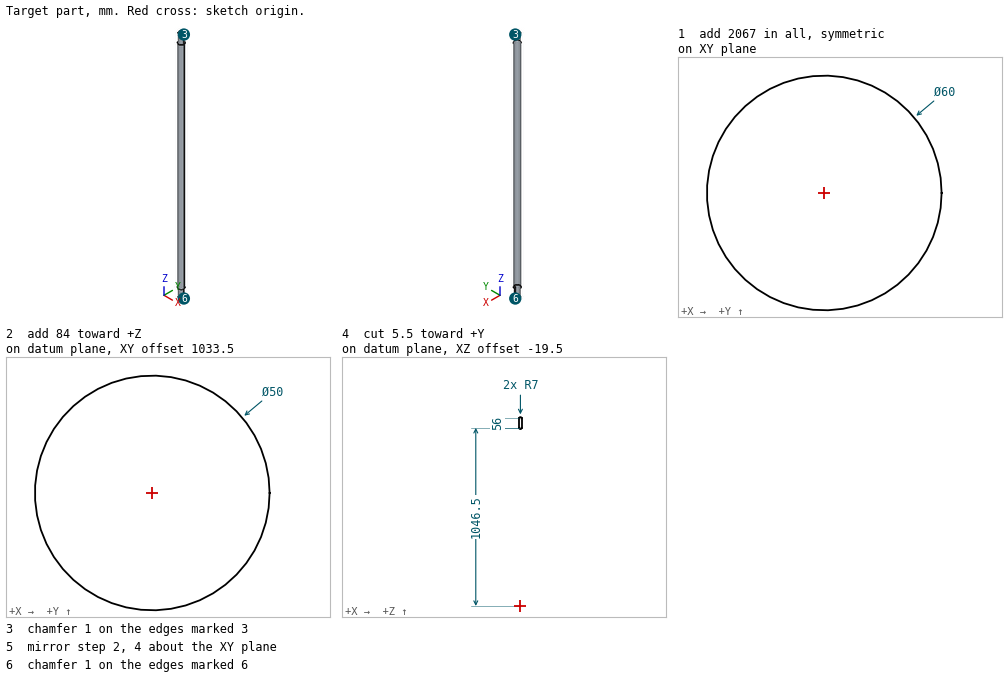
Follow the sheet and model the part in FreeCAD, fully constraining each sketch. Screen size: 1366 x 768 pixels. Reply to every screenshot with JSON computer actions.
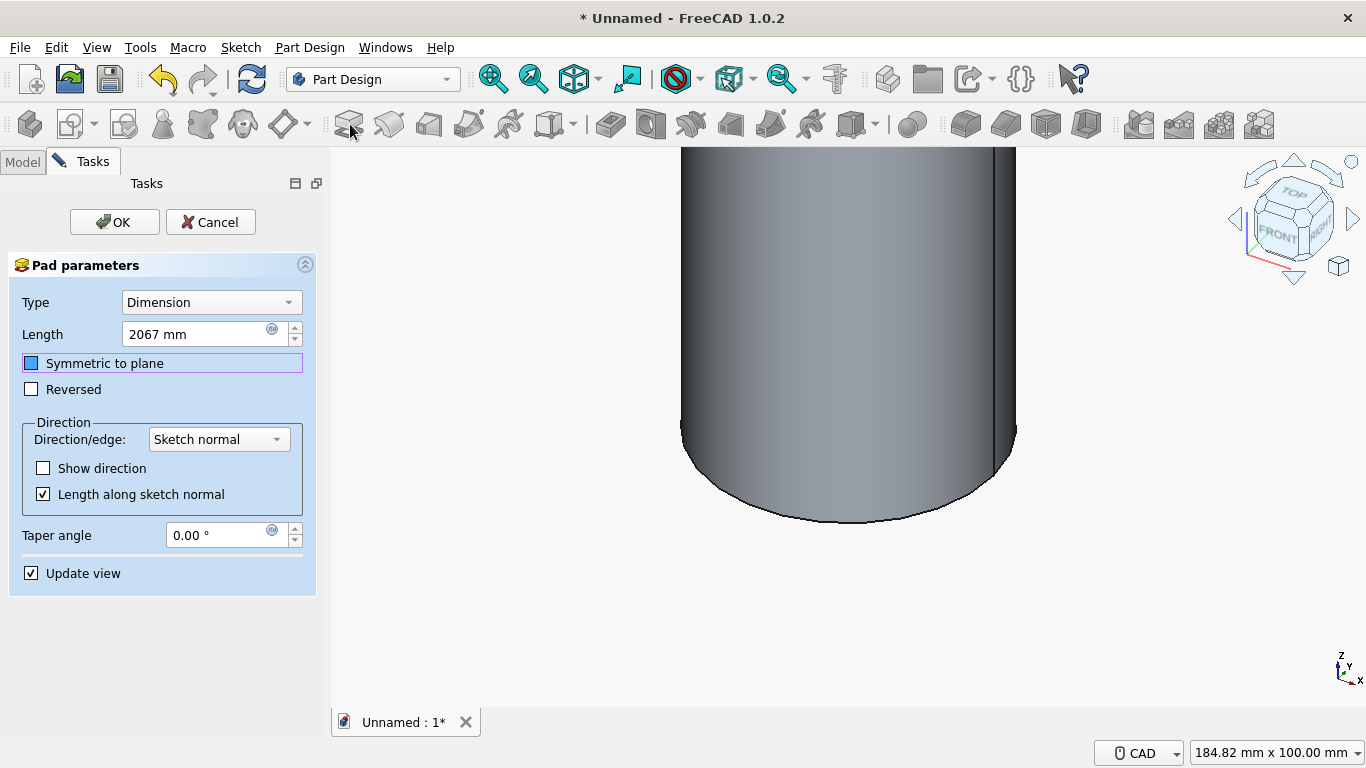
{"action": "left_click", "coordinate": [30, 363]}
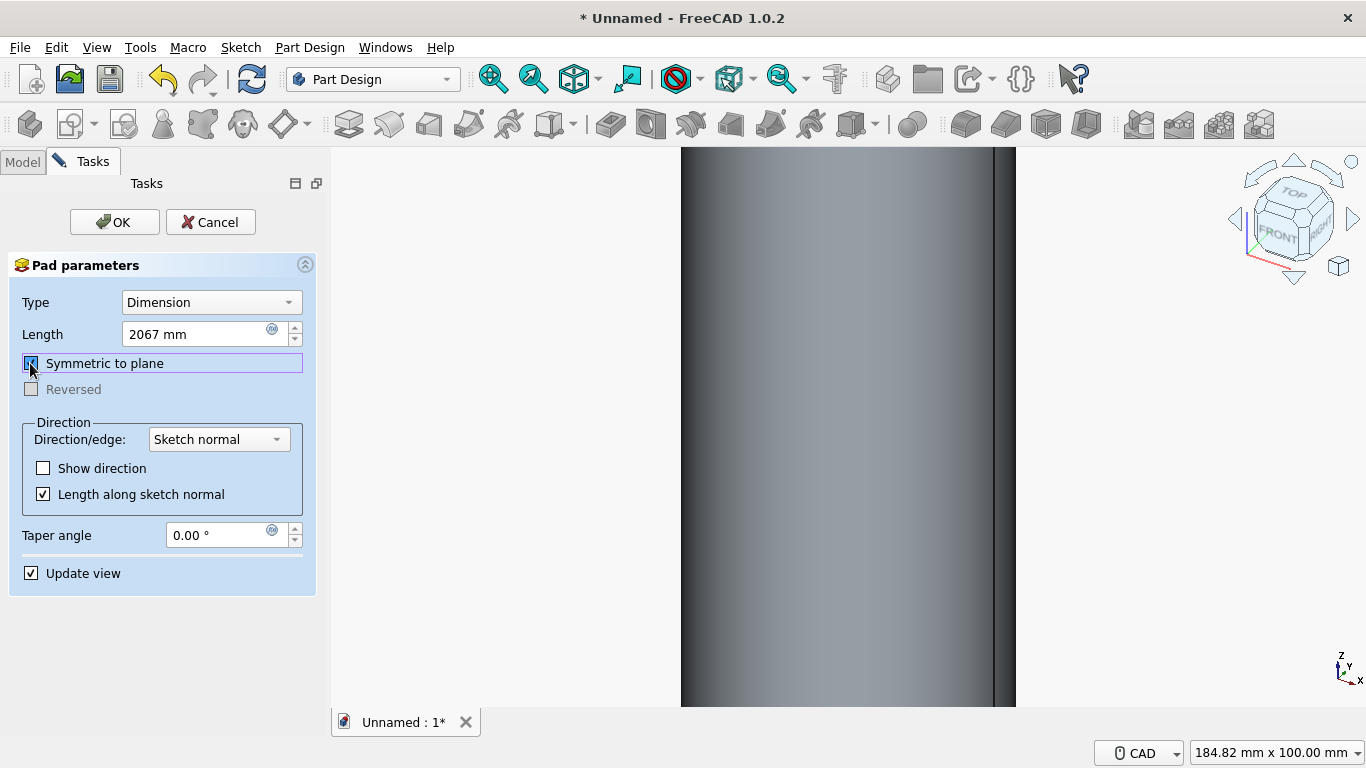
{"action": "left_click", "coordinate": [115, 222]}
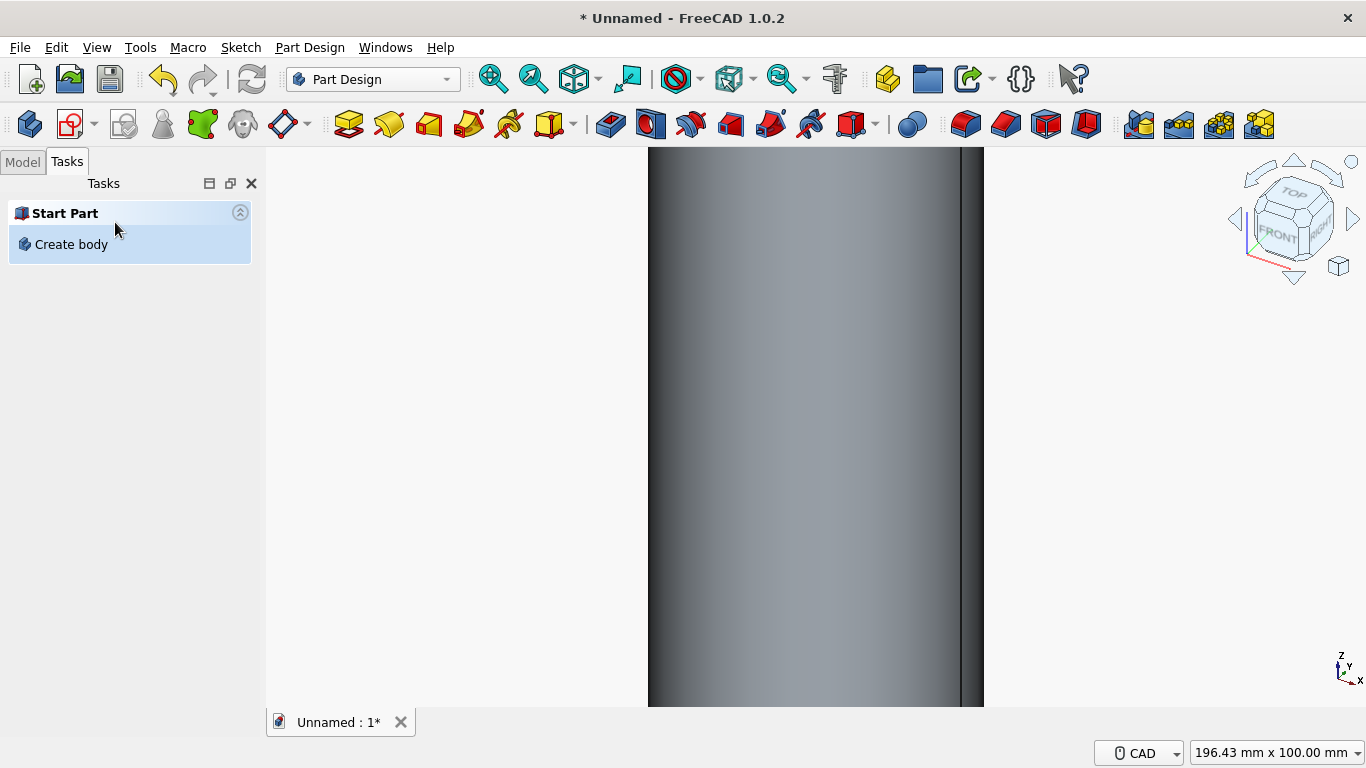
{"action": "left_click", "coordinate": [494, 80]}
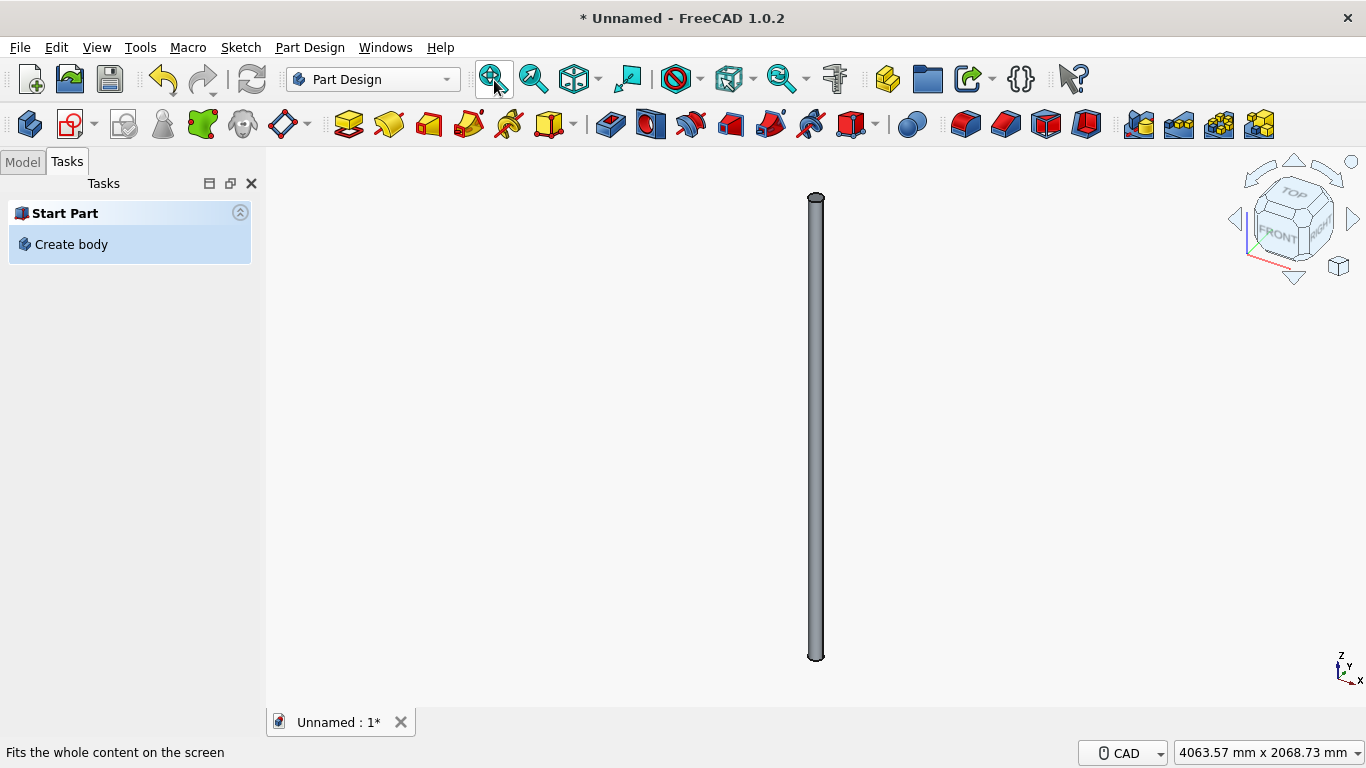
{"action": "key", "text": "0"}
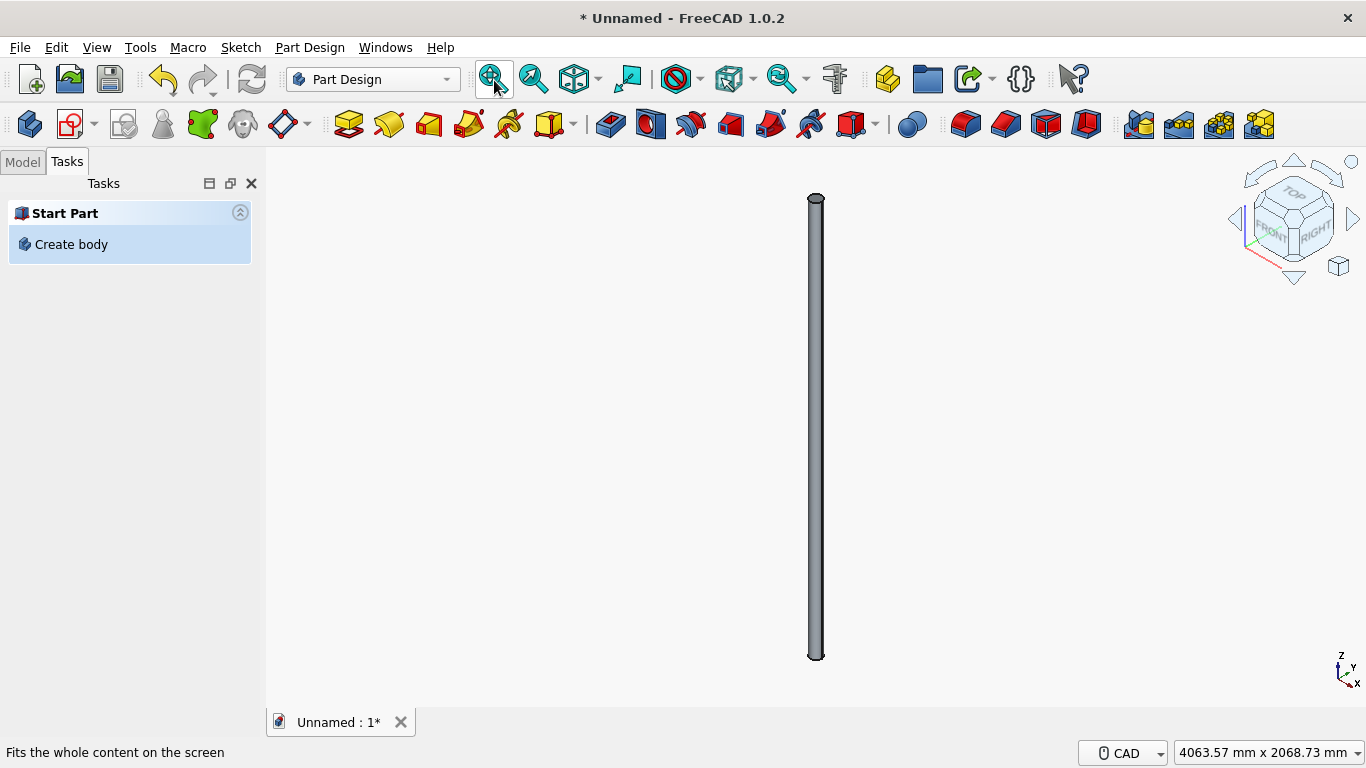
{"action": "key", "text": "2"}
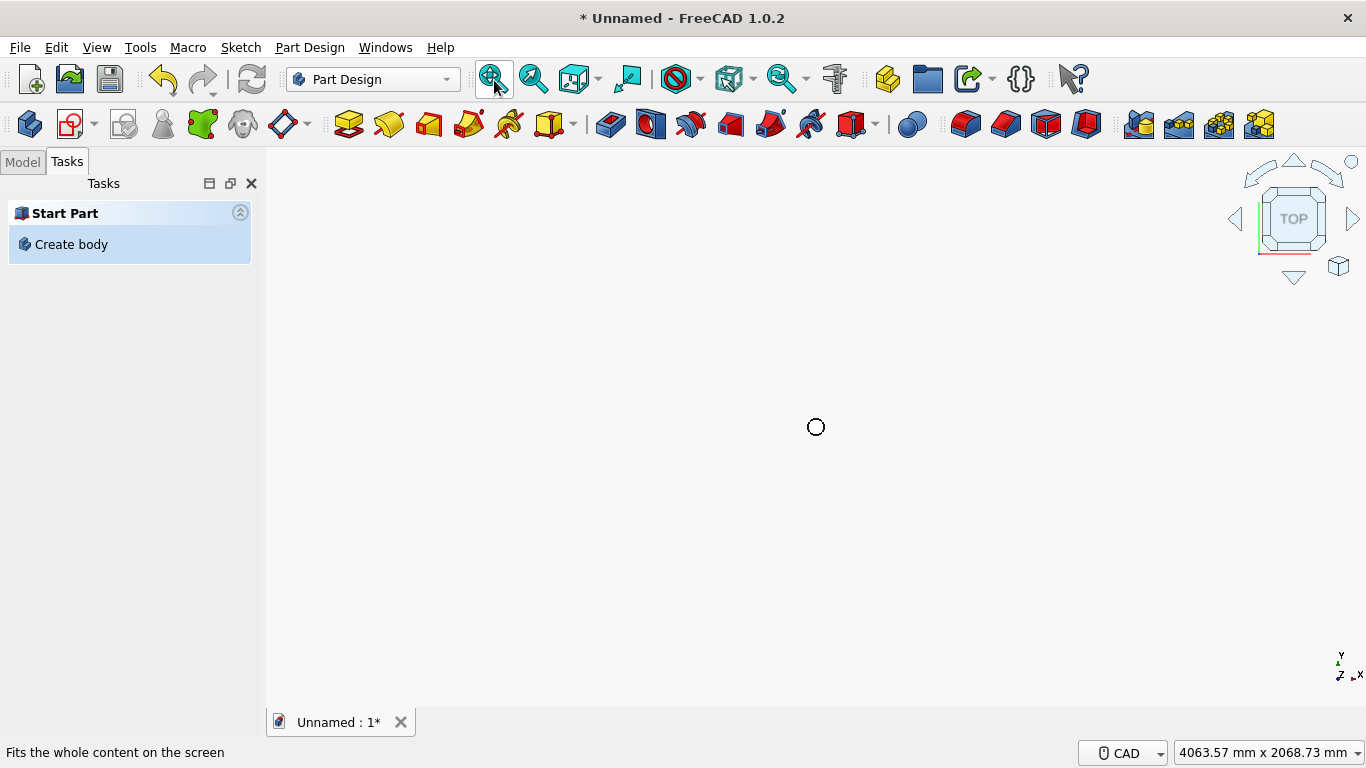
{"action": "left_click", "coordinate": [494, 80]}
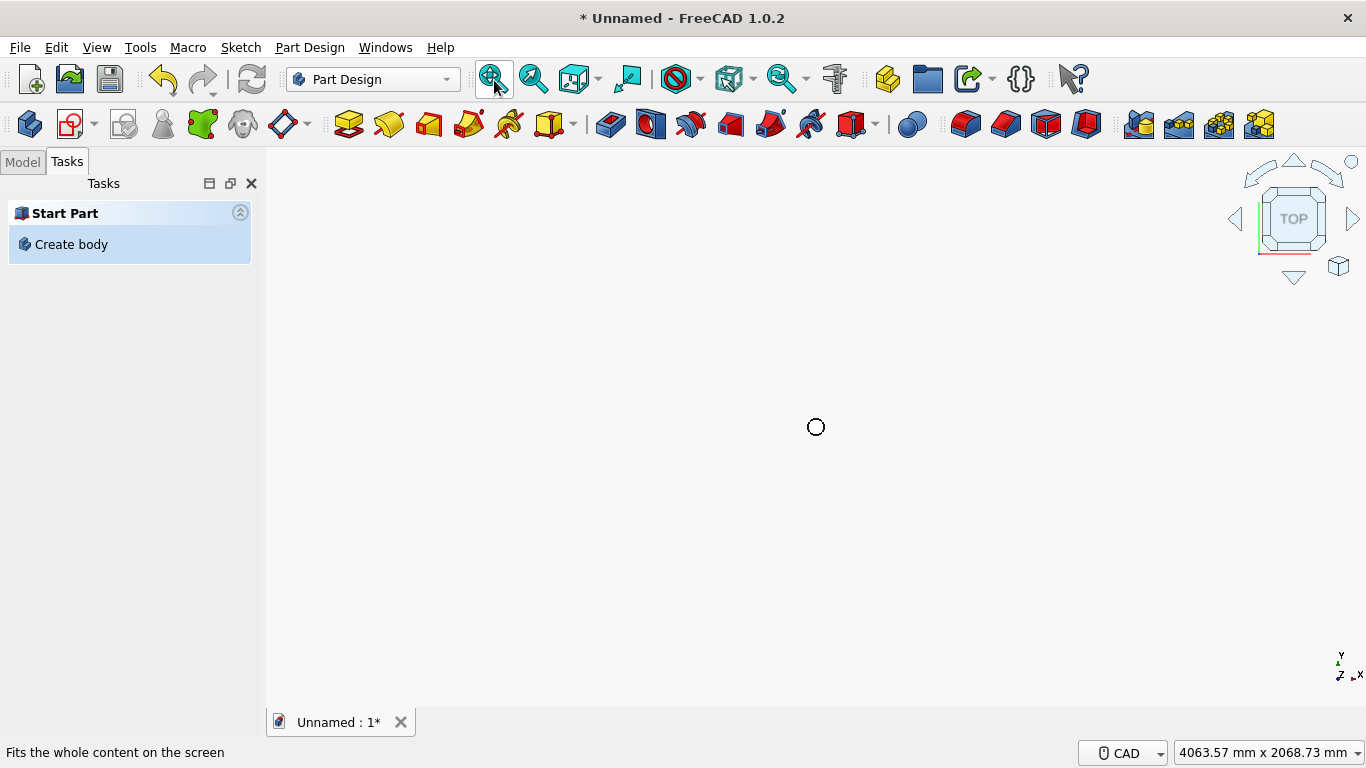
{"action": "key", "text": "1"}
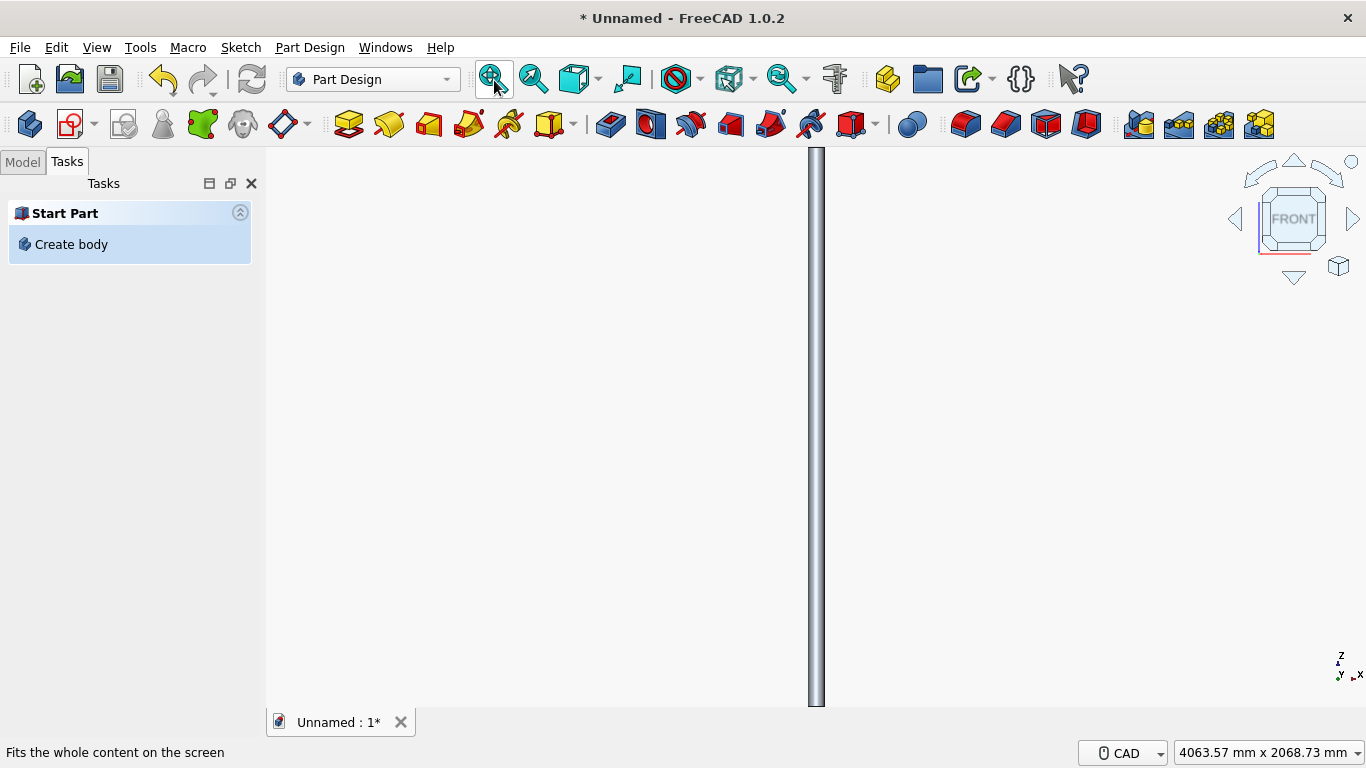
{"action": "left_click", "coordinate": [494, 80]}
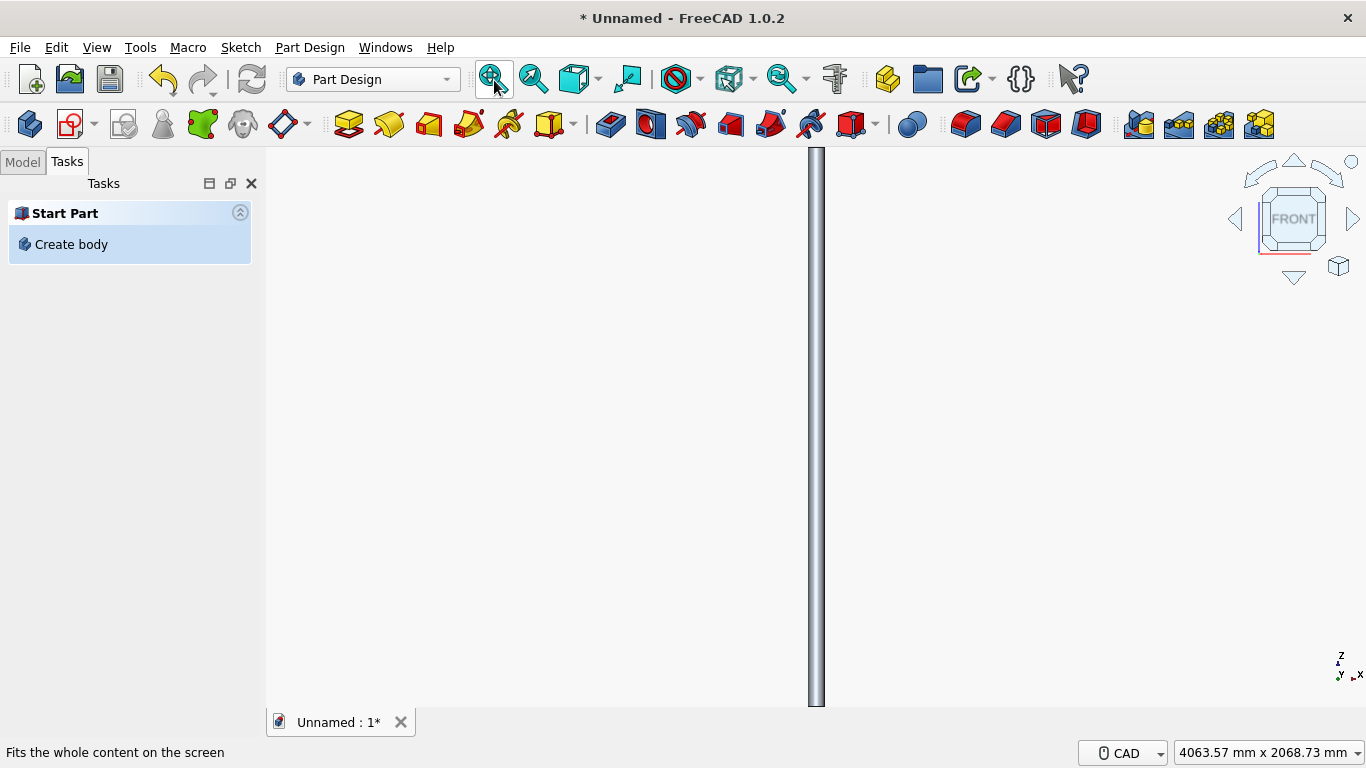
{"action": "left_click", "coordinate": [23, 161]}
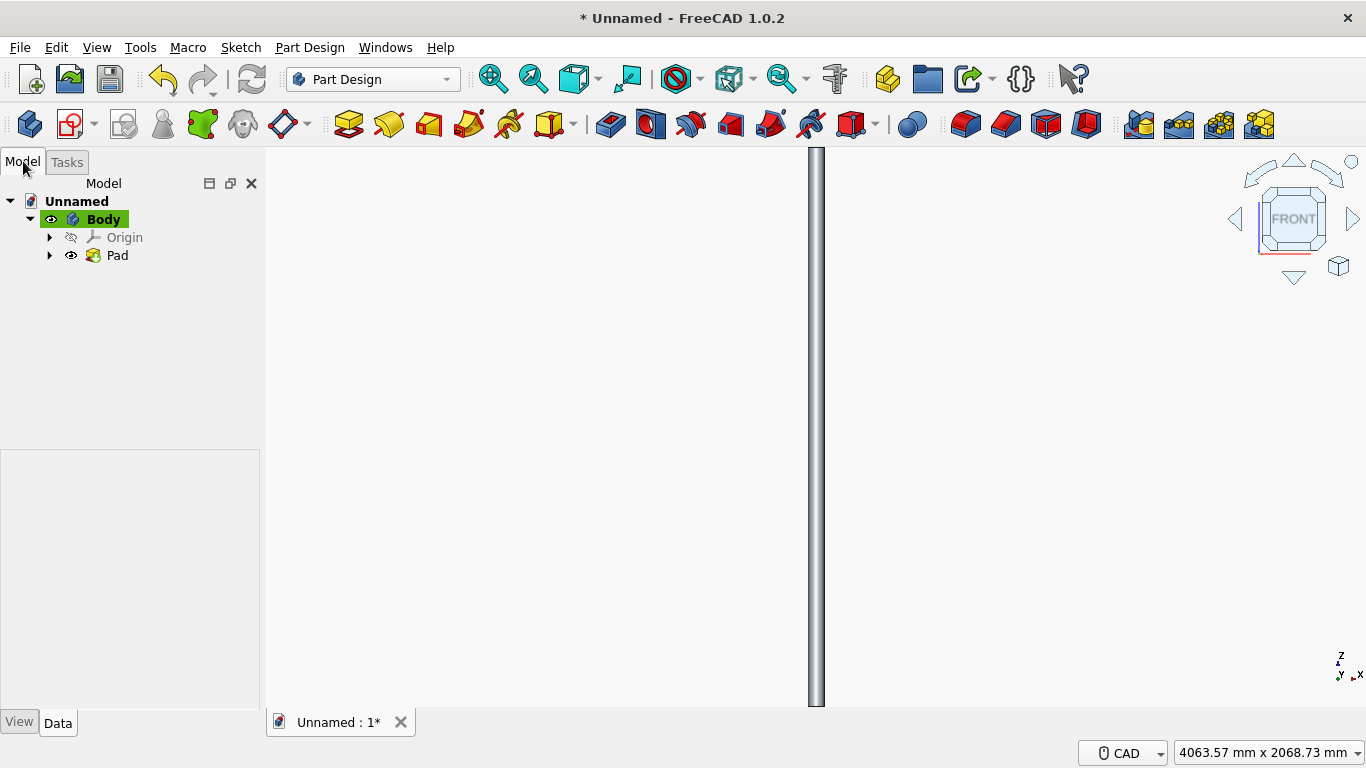
{"action": "left_click", "coordinate": [50, 237]}